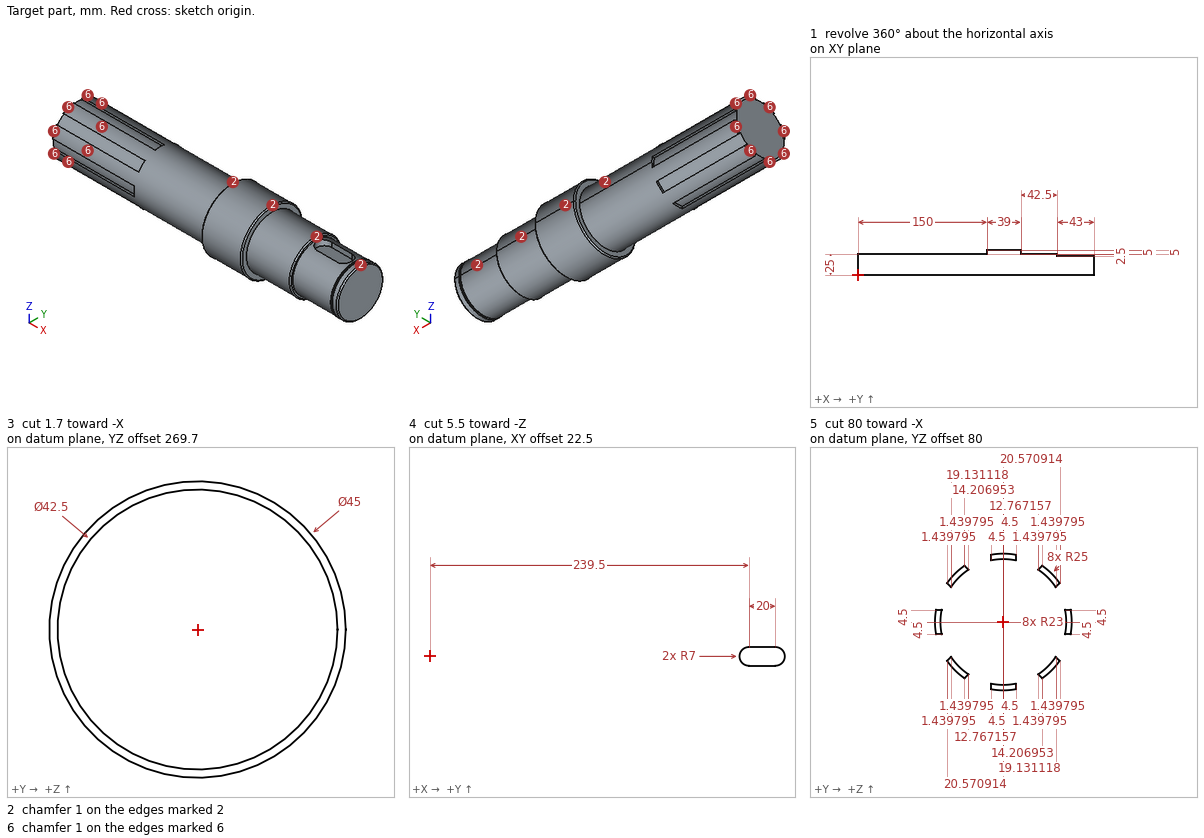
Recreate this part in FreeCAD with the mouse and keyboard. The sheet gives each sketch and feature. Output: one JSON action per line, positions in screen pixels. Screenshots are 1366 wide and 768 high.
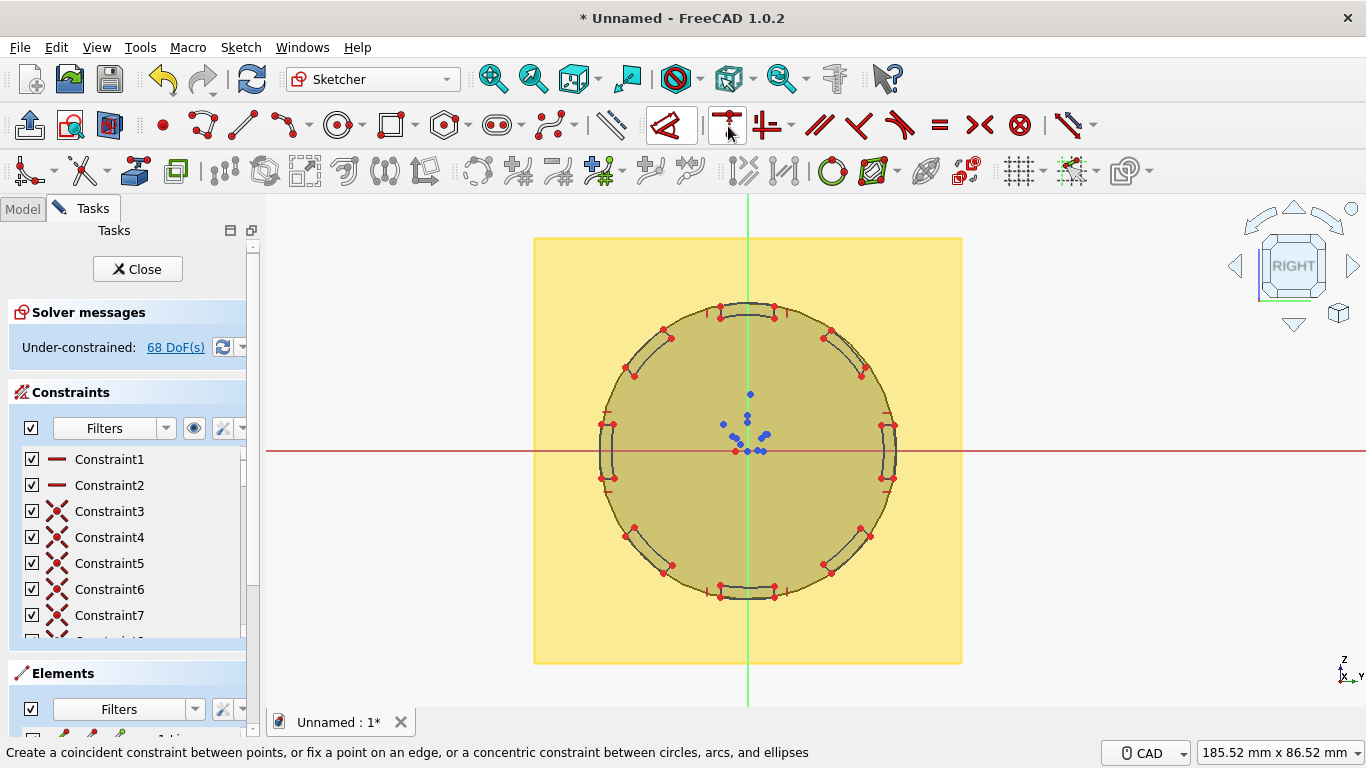
{"action": "left_click", "coordinate": [883, 463]}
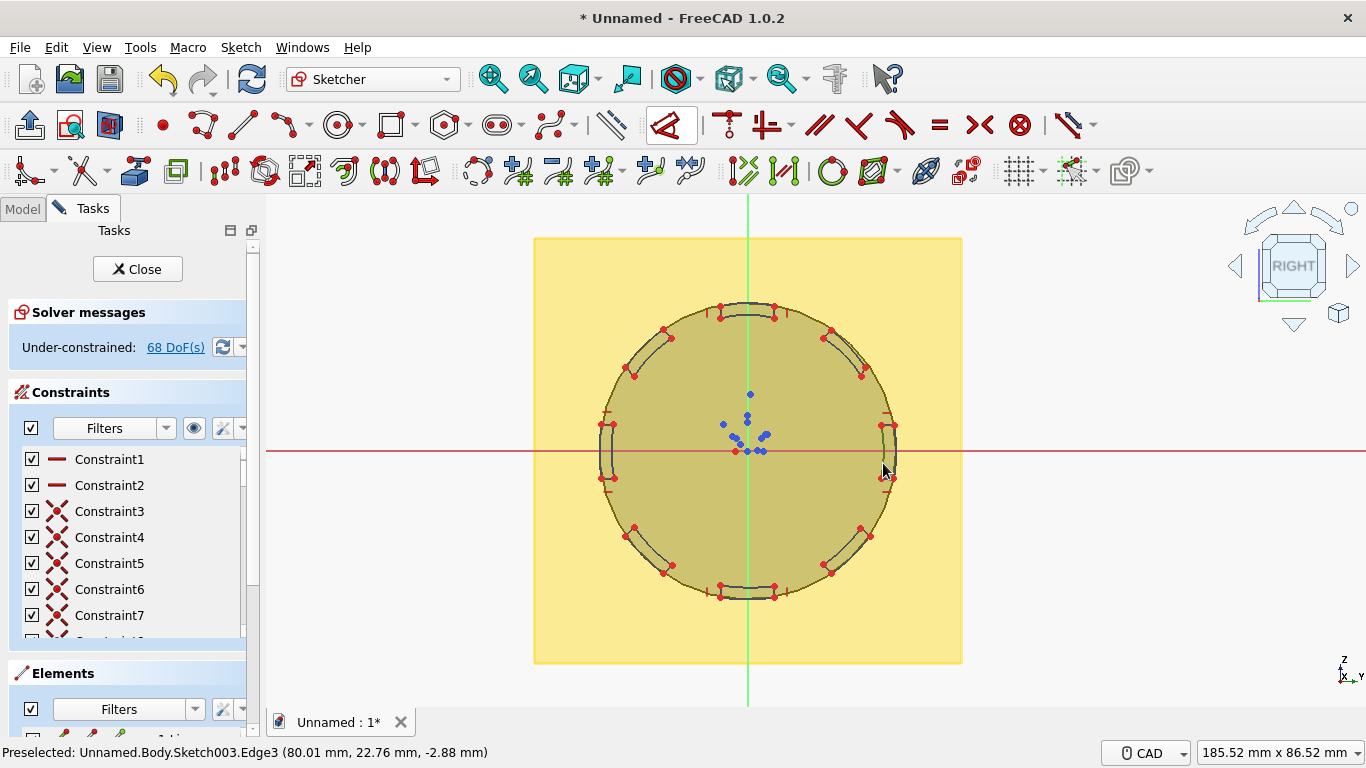
{"action": "scroll", "coordinate": [836, 348], "scroll_direction": "up", "scroll_amount": 2}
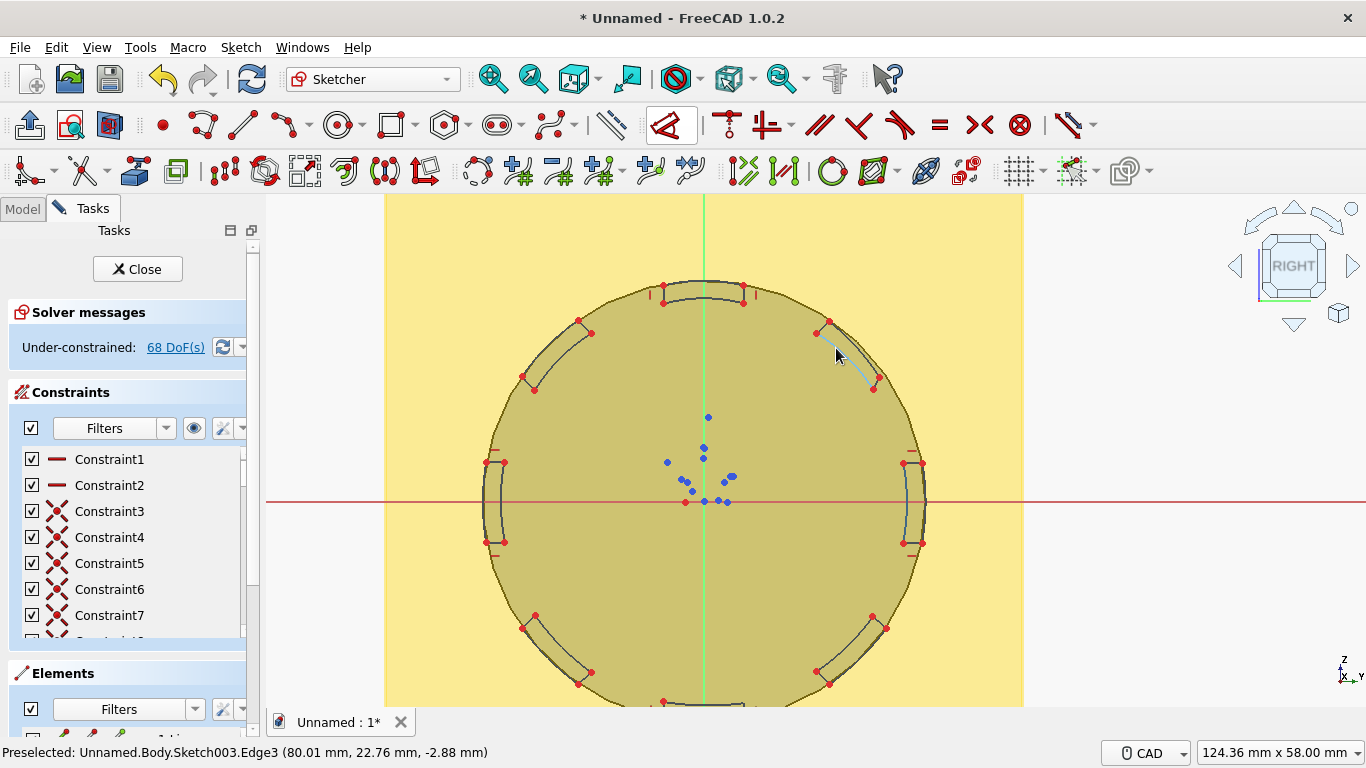
{"action": "left_click", "coordinate": [836, 347]}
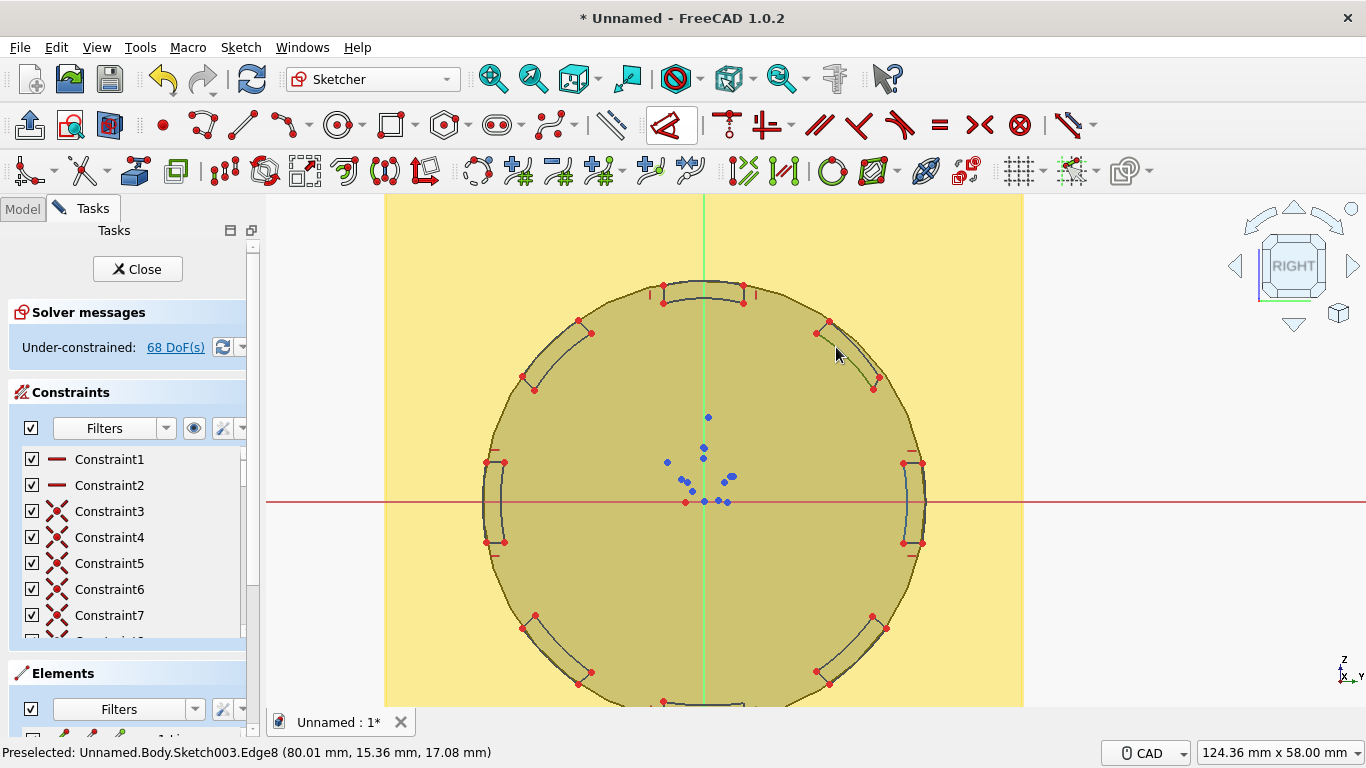
{"action": "key", "text": "c"}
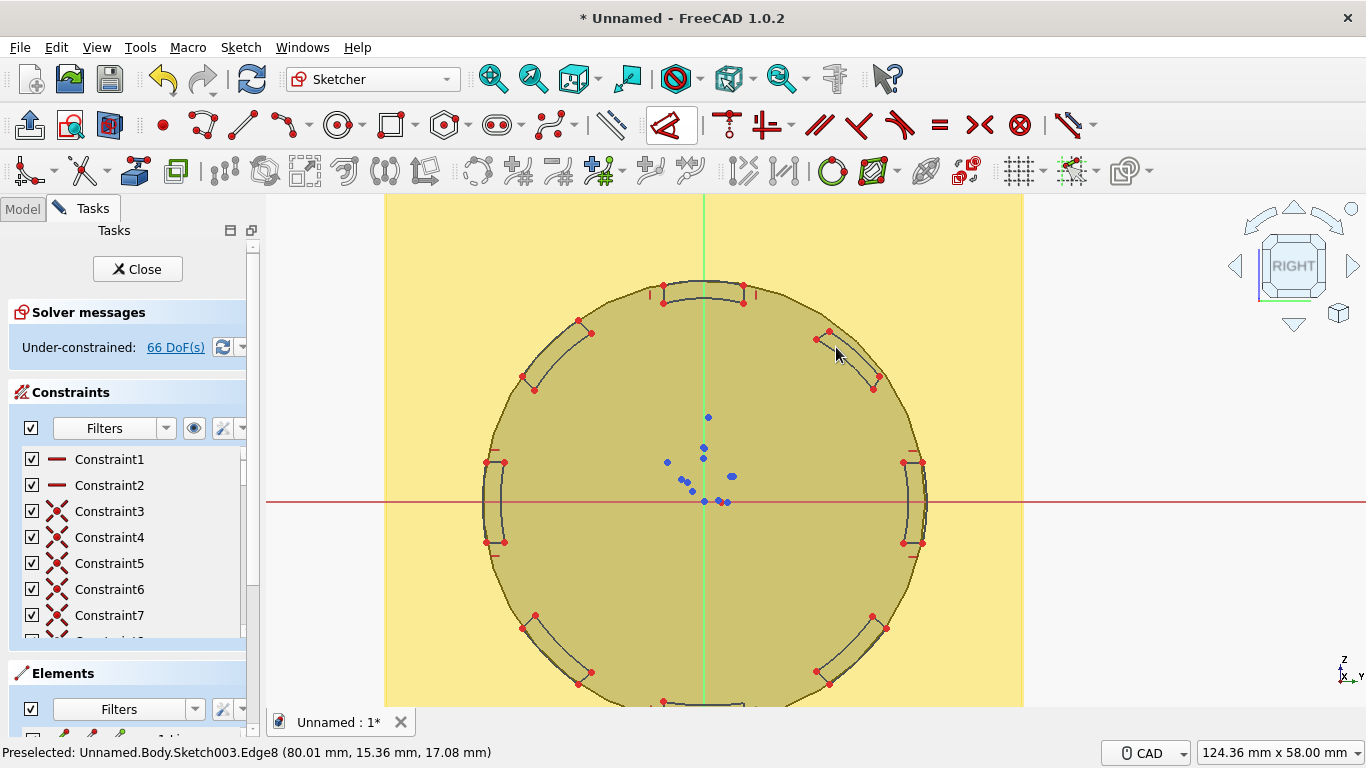
{"action": "left_click", "coordinate": [907, 519]}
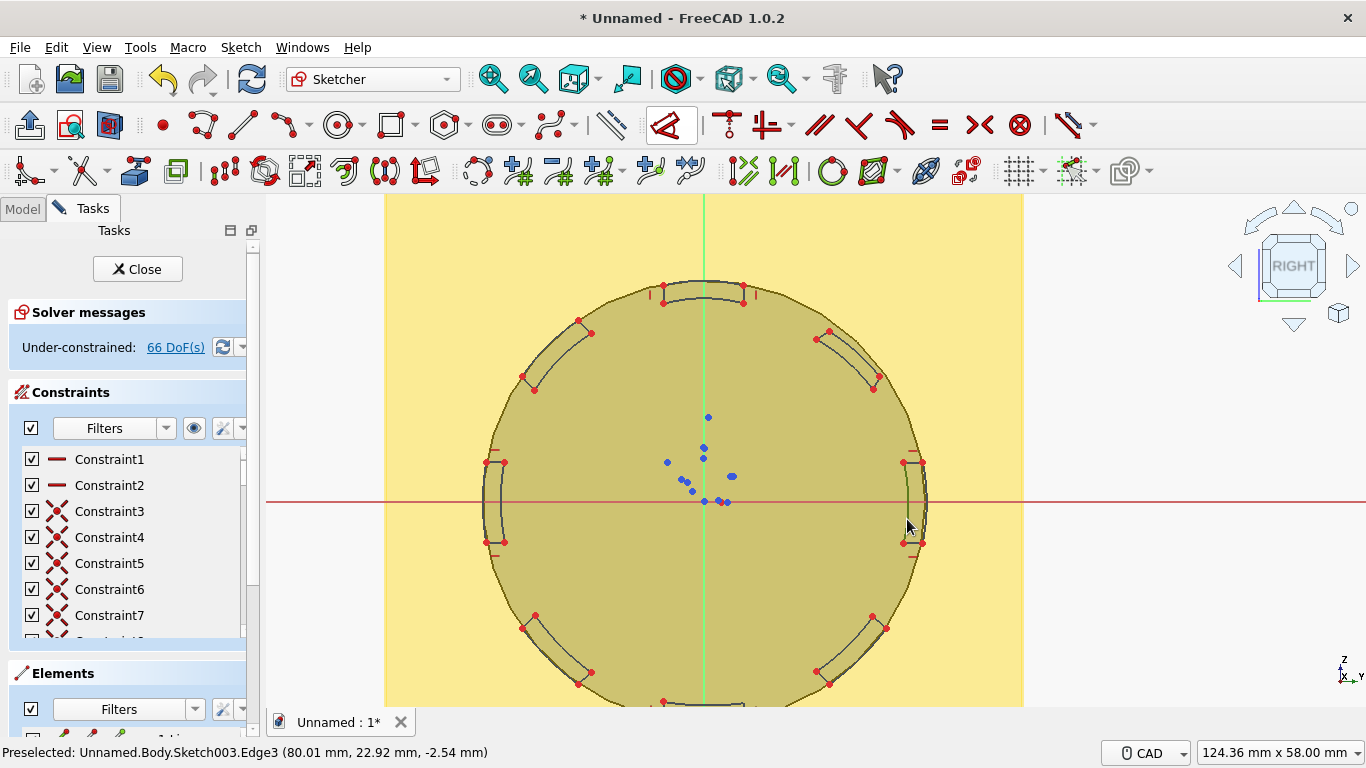
{"action": "left_click", "coordinate": [720, 281]}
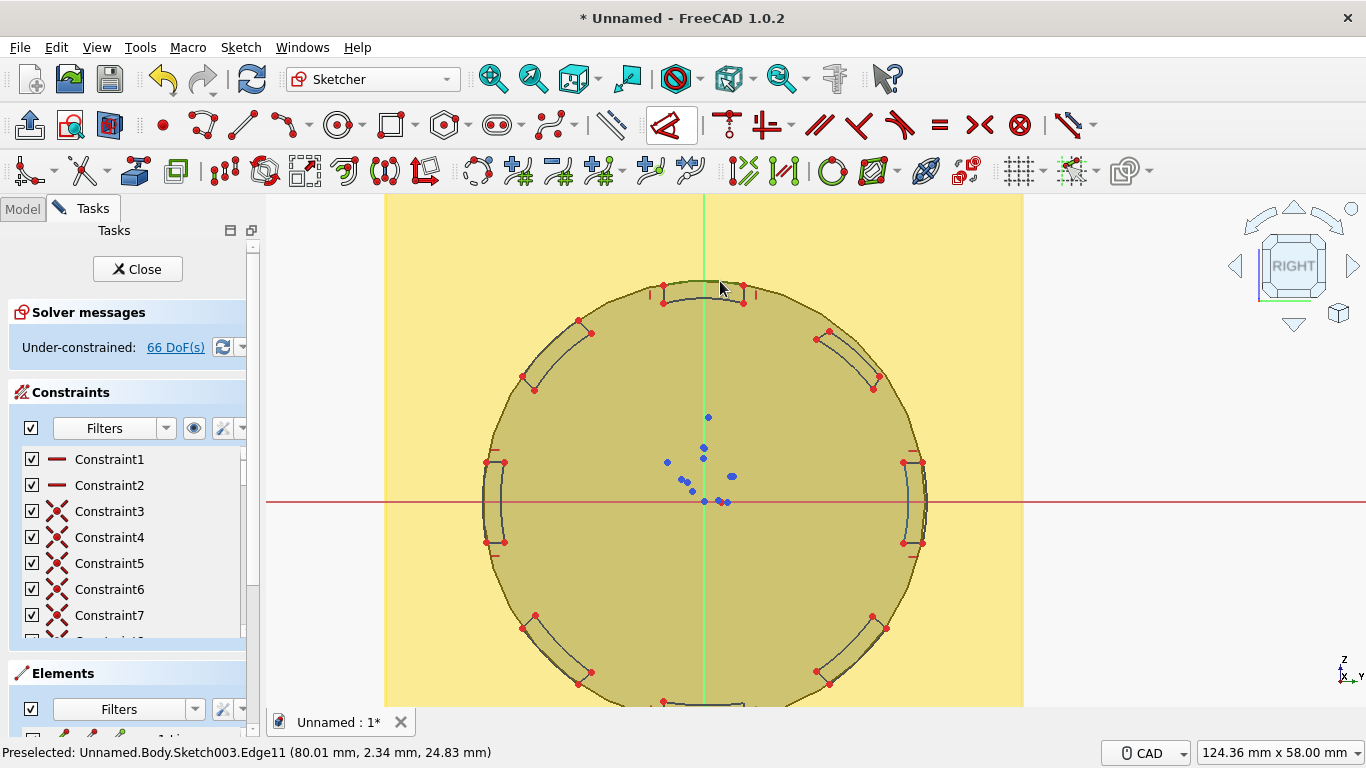
{"action": "left_click", "coordinate": [728, 126]}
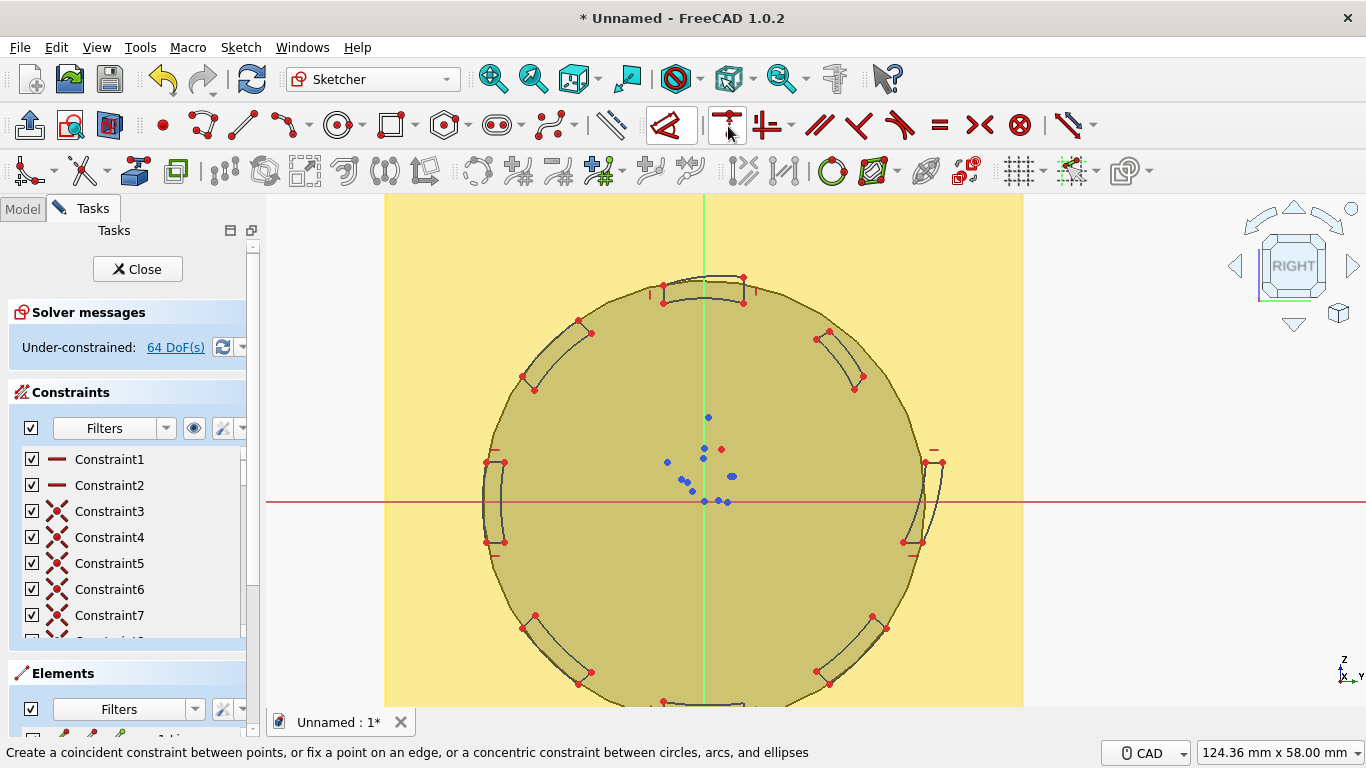
{"action": "left_click", "coordinate": [914, 520]}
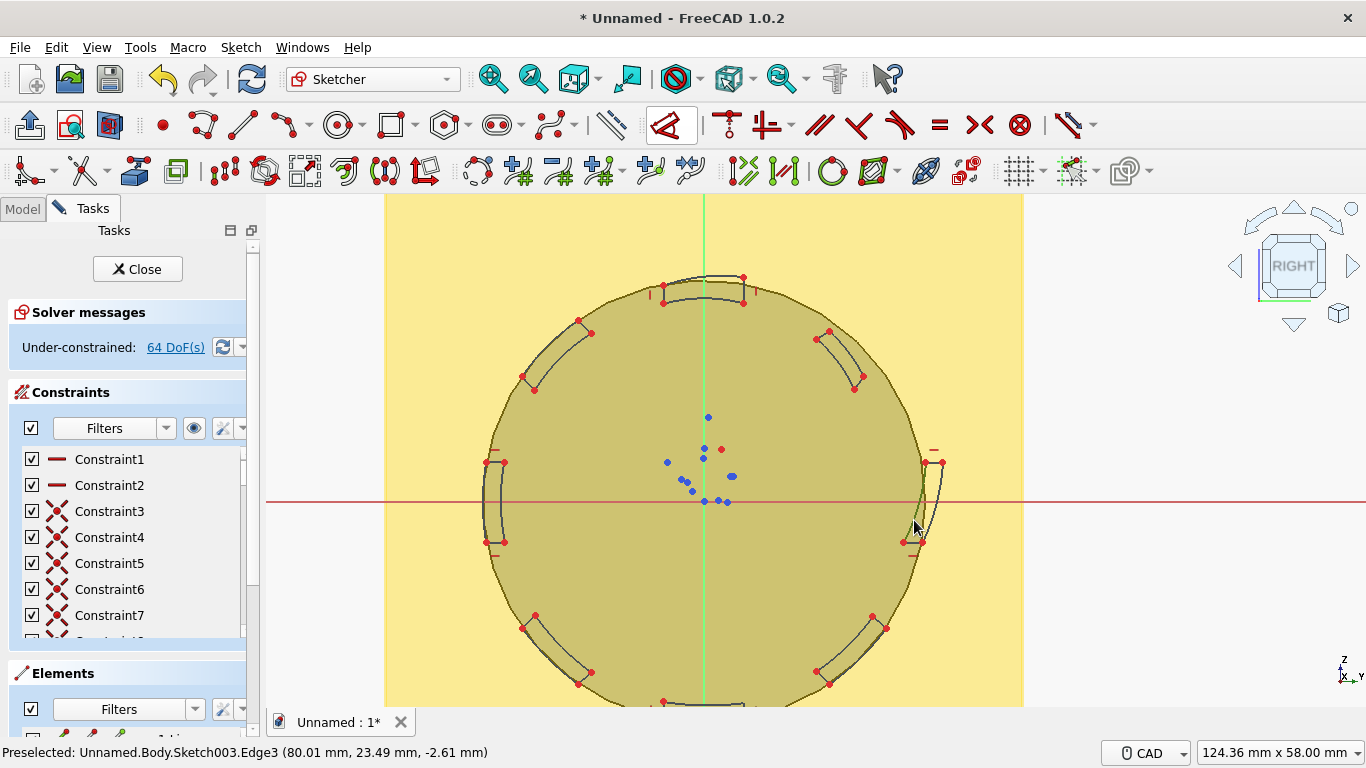
{"action": "left_click", "coordinate": [720, 299]}